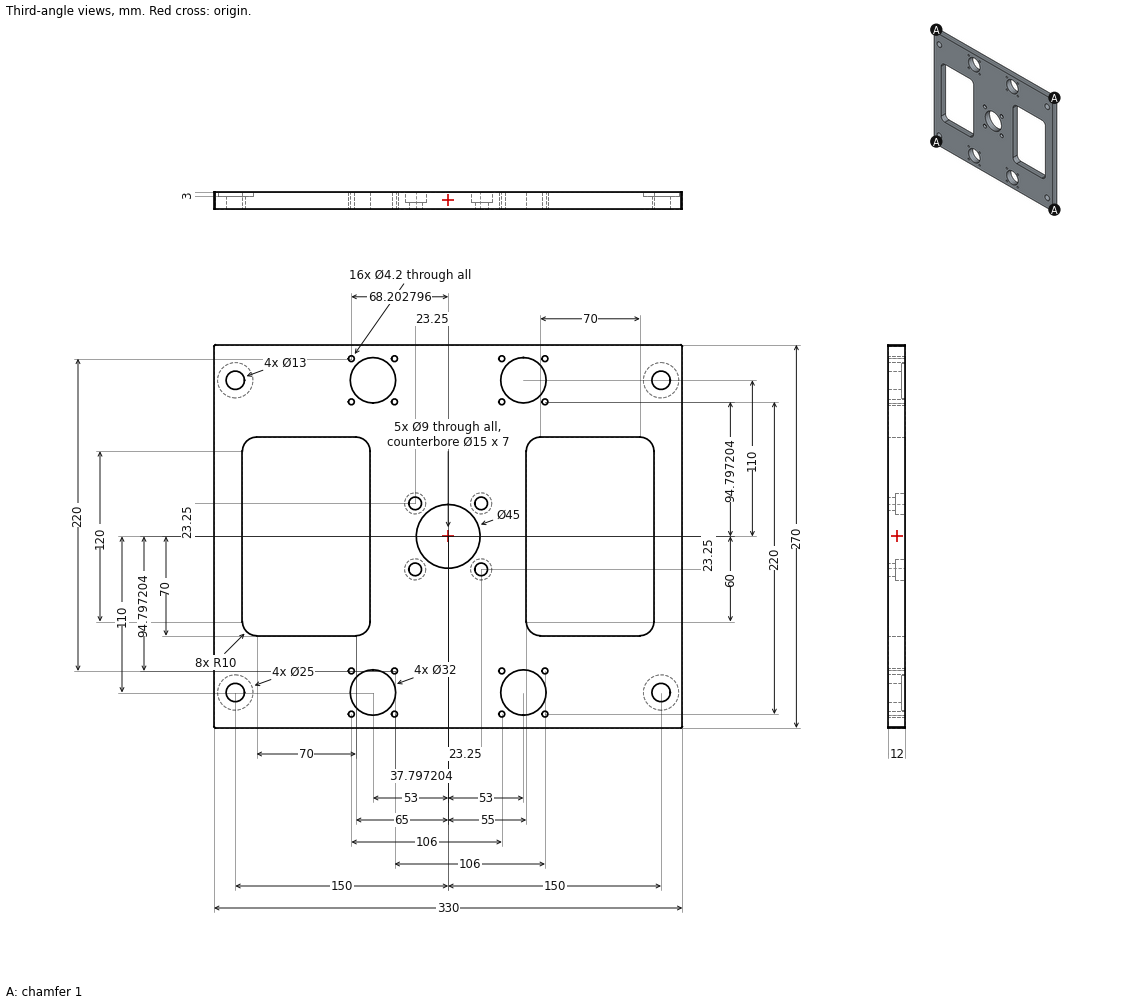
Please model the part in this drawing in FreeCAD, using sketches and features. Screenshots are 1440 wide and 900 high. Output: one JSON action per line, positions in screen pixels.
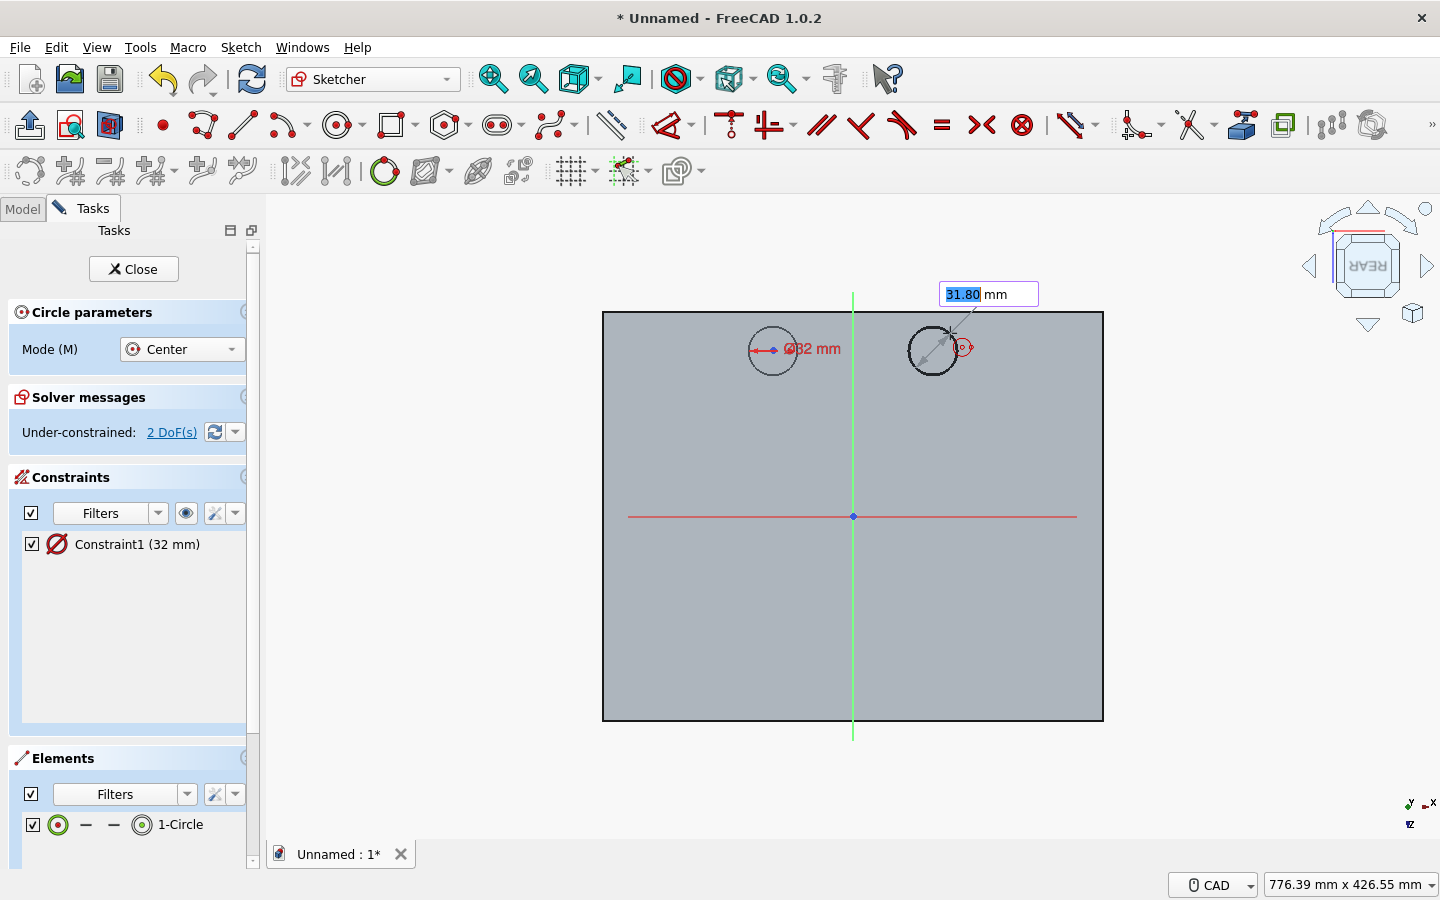
{"action": "type", "text": "32"}
{"action": "key", "text": "Return"}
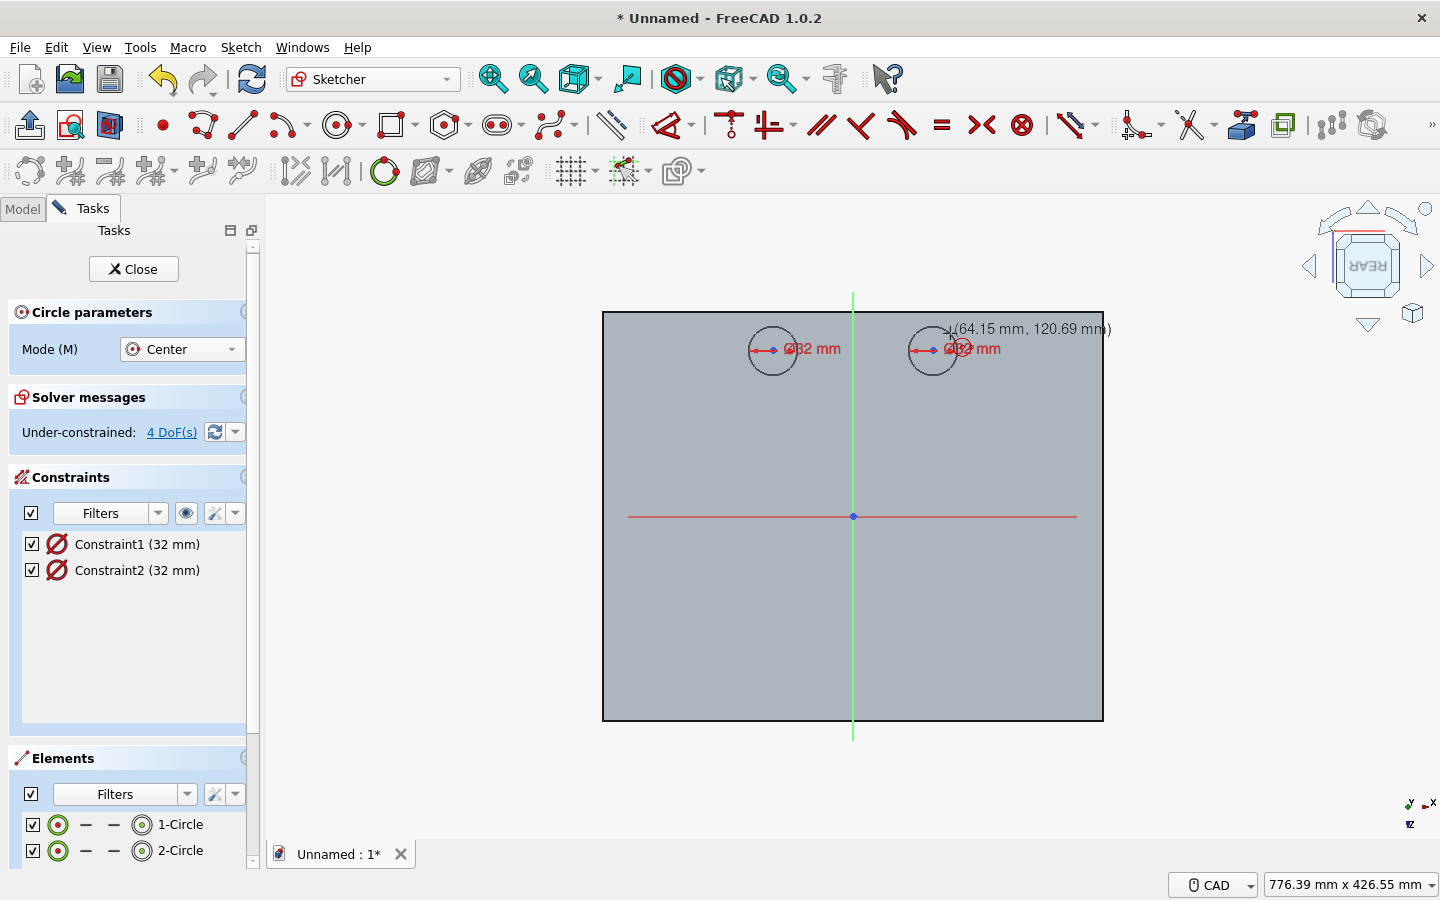
{"action": "left_click", "coordinate": [933, 683]}
{"action": "mouse_move", "coordinate": [950, 666]}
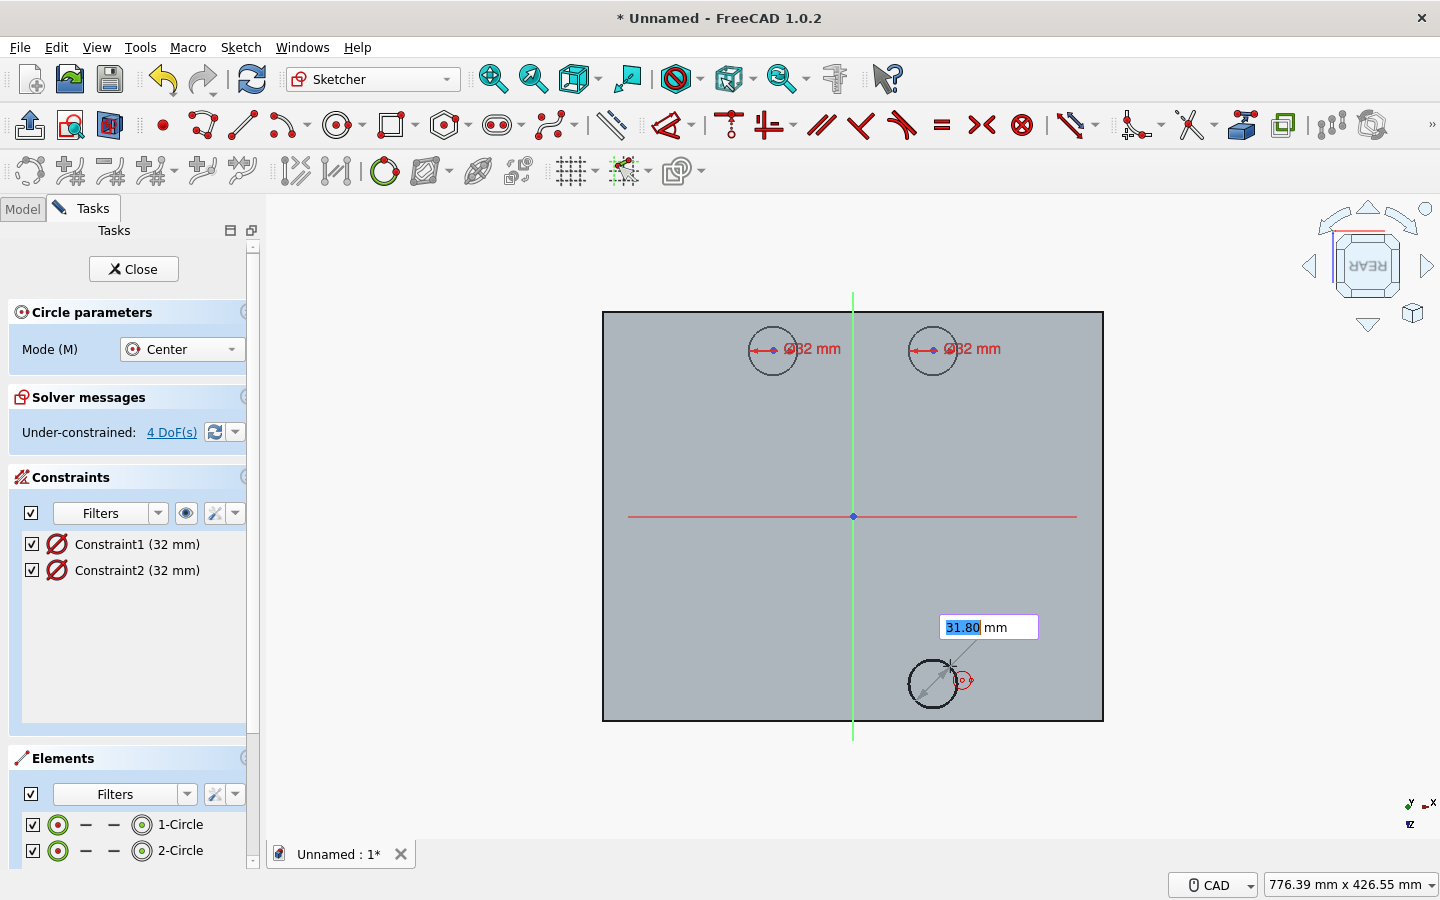
{"action": "type", "text": "32"}
{"action": "key", "text": "Return"}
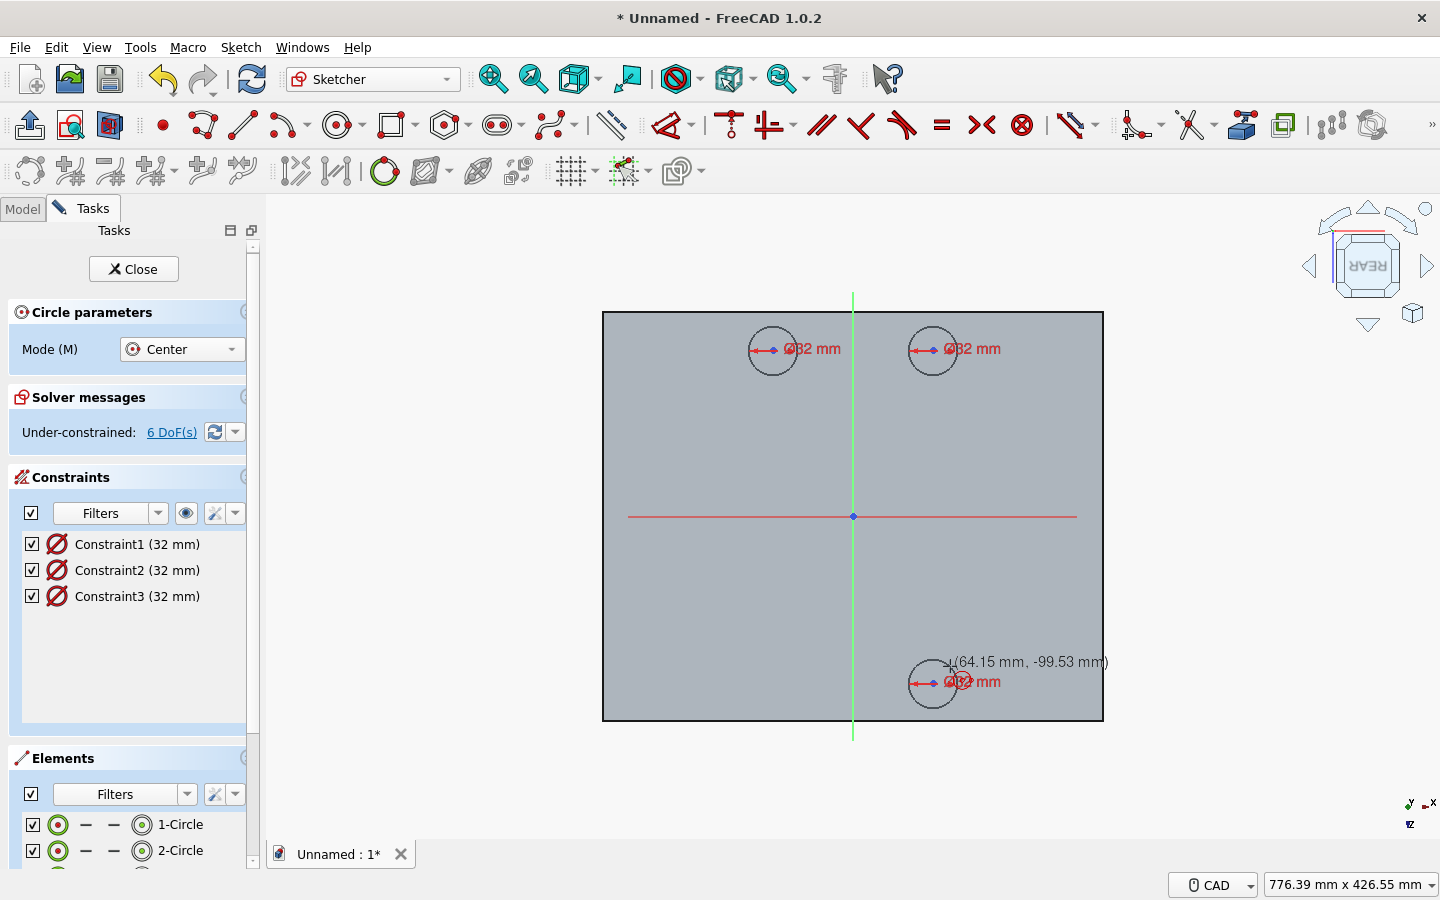
{"action": "left_click", "coordinate": [773, 683]}
{"action": "mouse_move", "coordinate": [790, 666]}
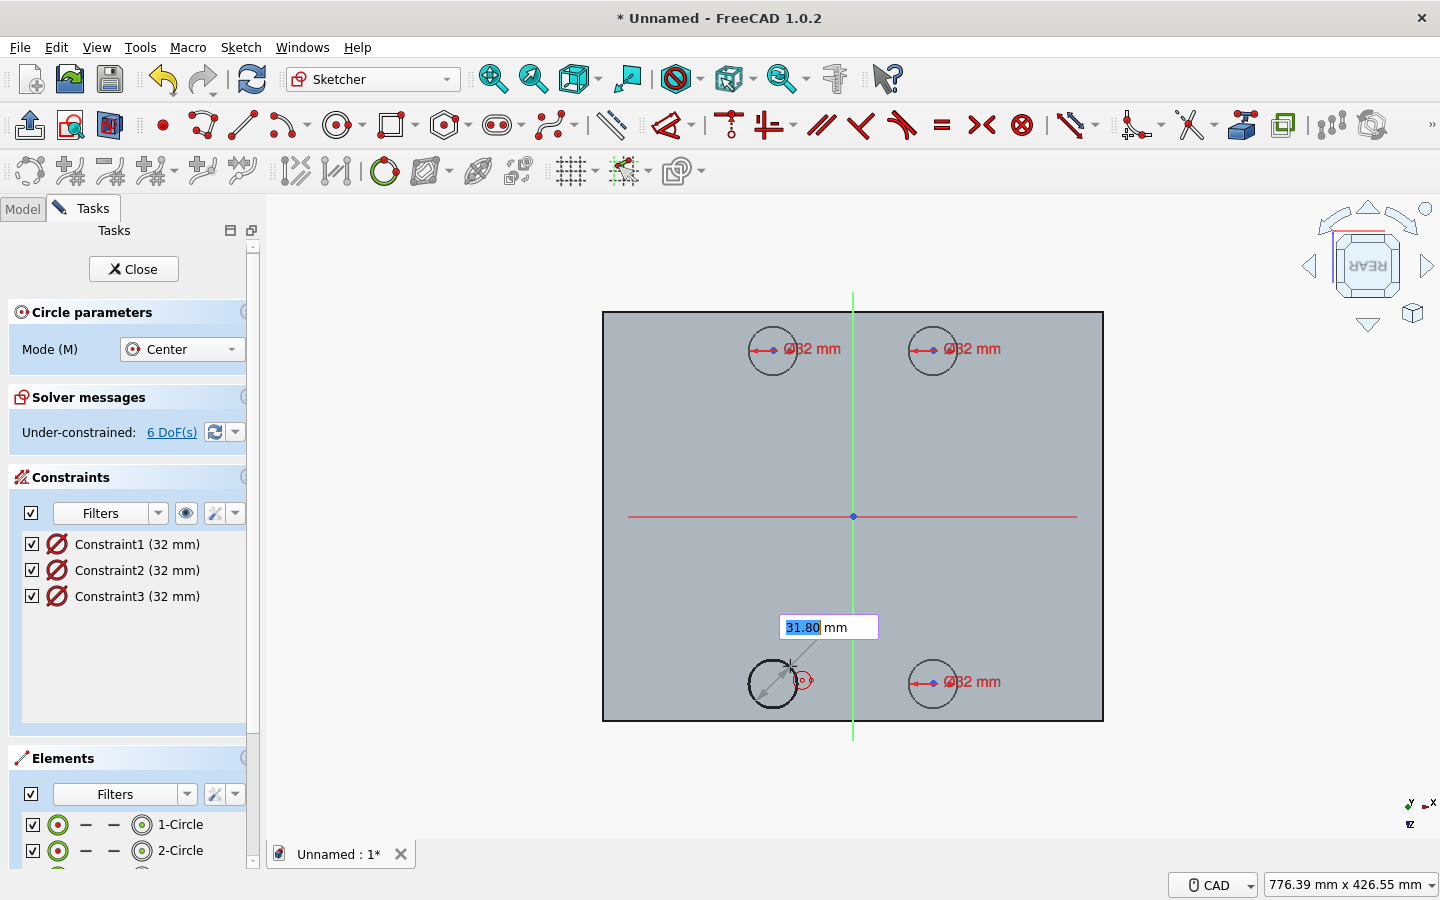
{"action": "type", "text": "32"}
{"action": "key", "text": "Return"}
{"action": "key", "text": "Escape"}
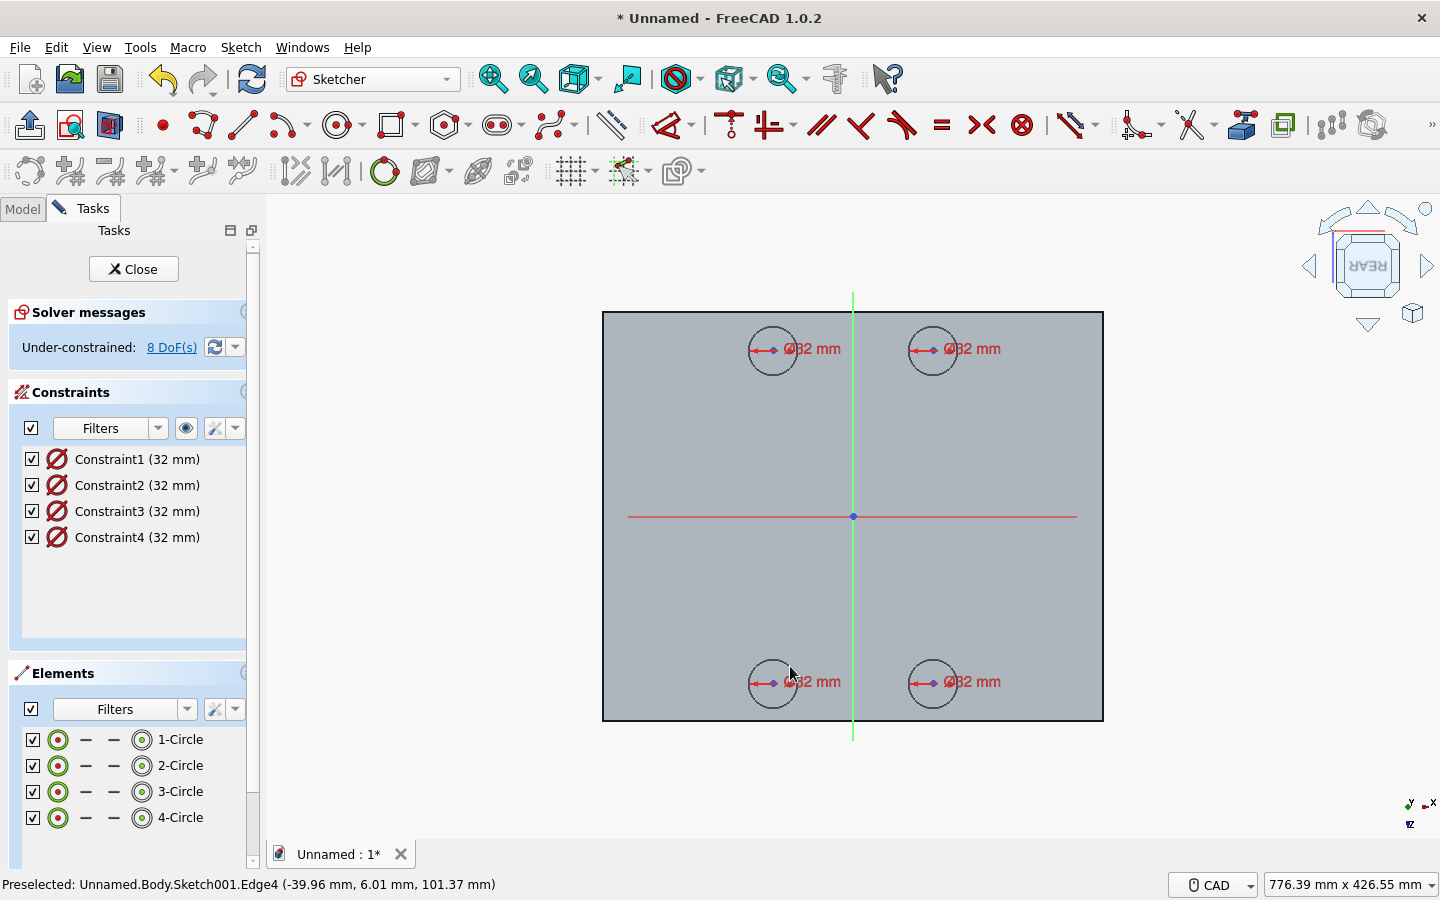
{"action": "left_click", "coordinate": [773, 351]}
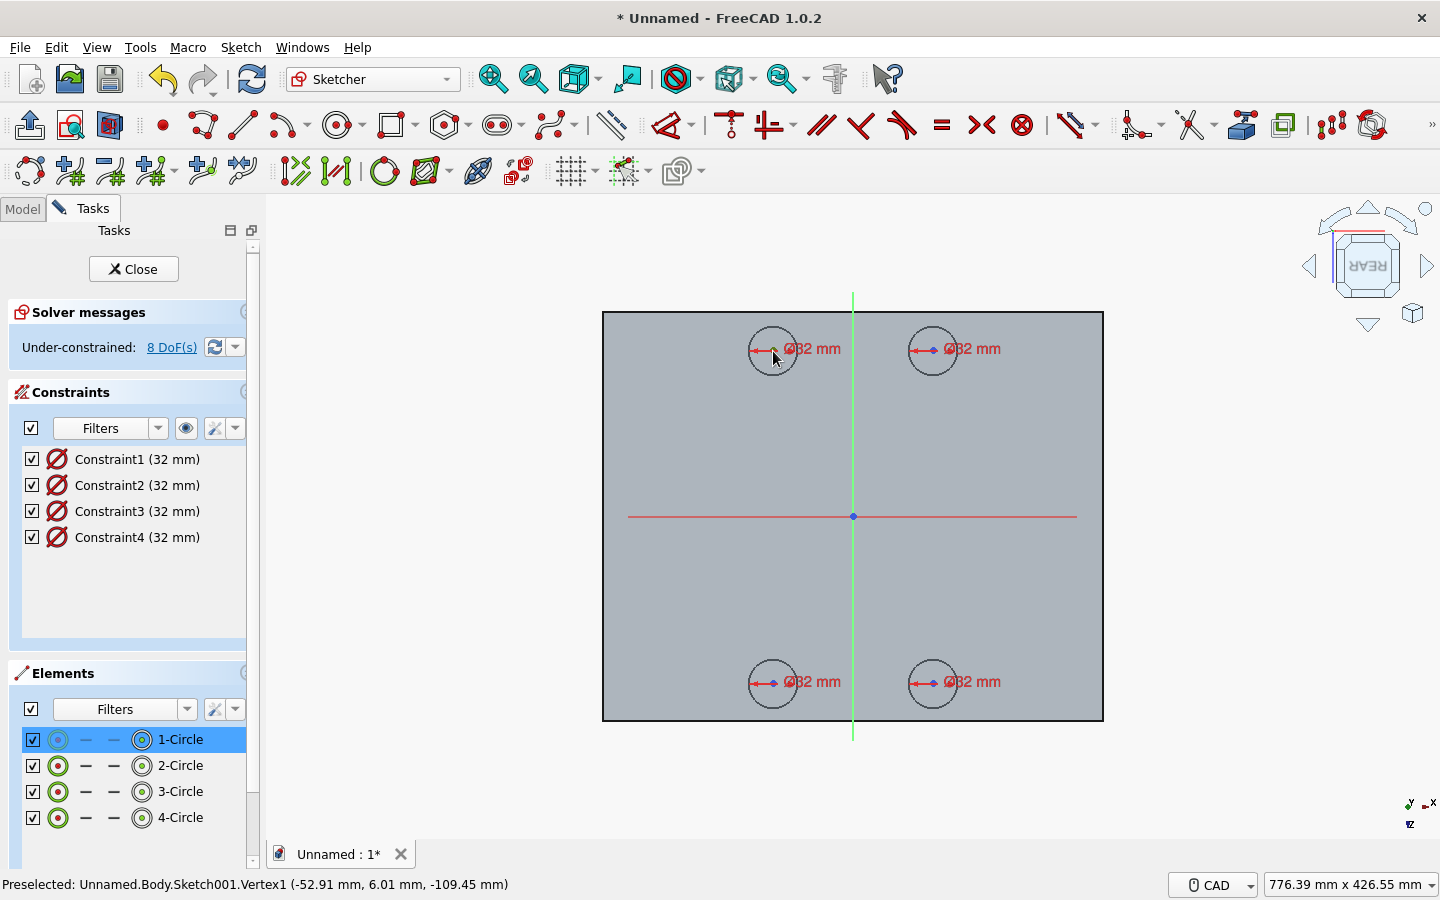
{"action": "left_click", "coordinate": [933, 351]}